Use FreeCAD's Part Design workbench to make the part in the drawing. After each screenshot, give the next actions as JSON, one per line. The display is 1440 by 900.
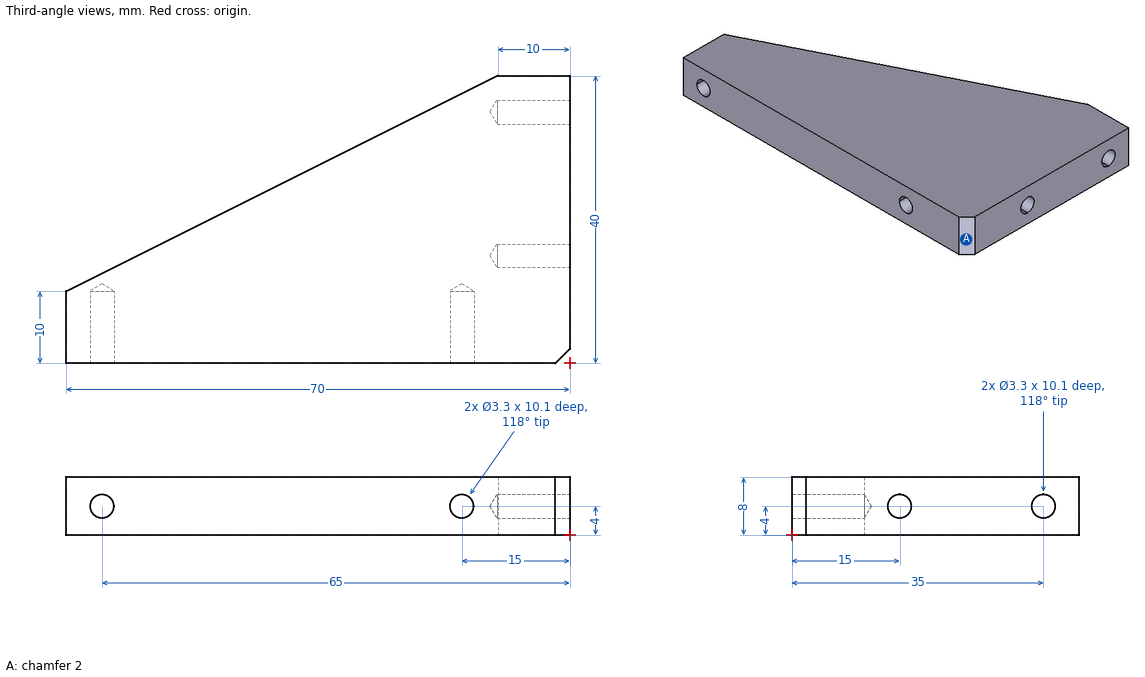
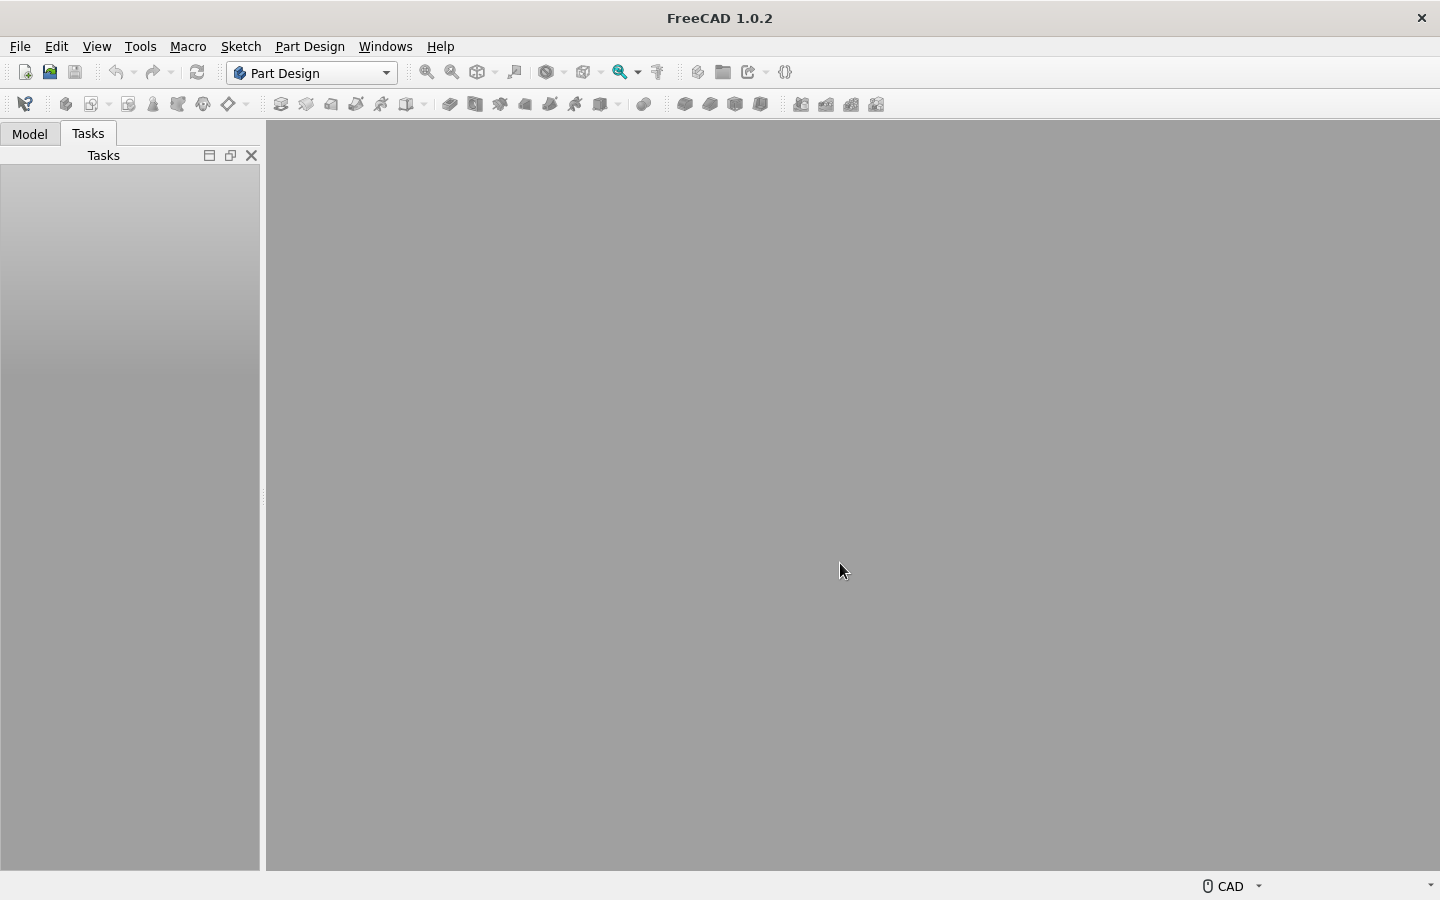
{"action": "key", "text": "ctrl+n"}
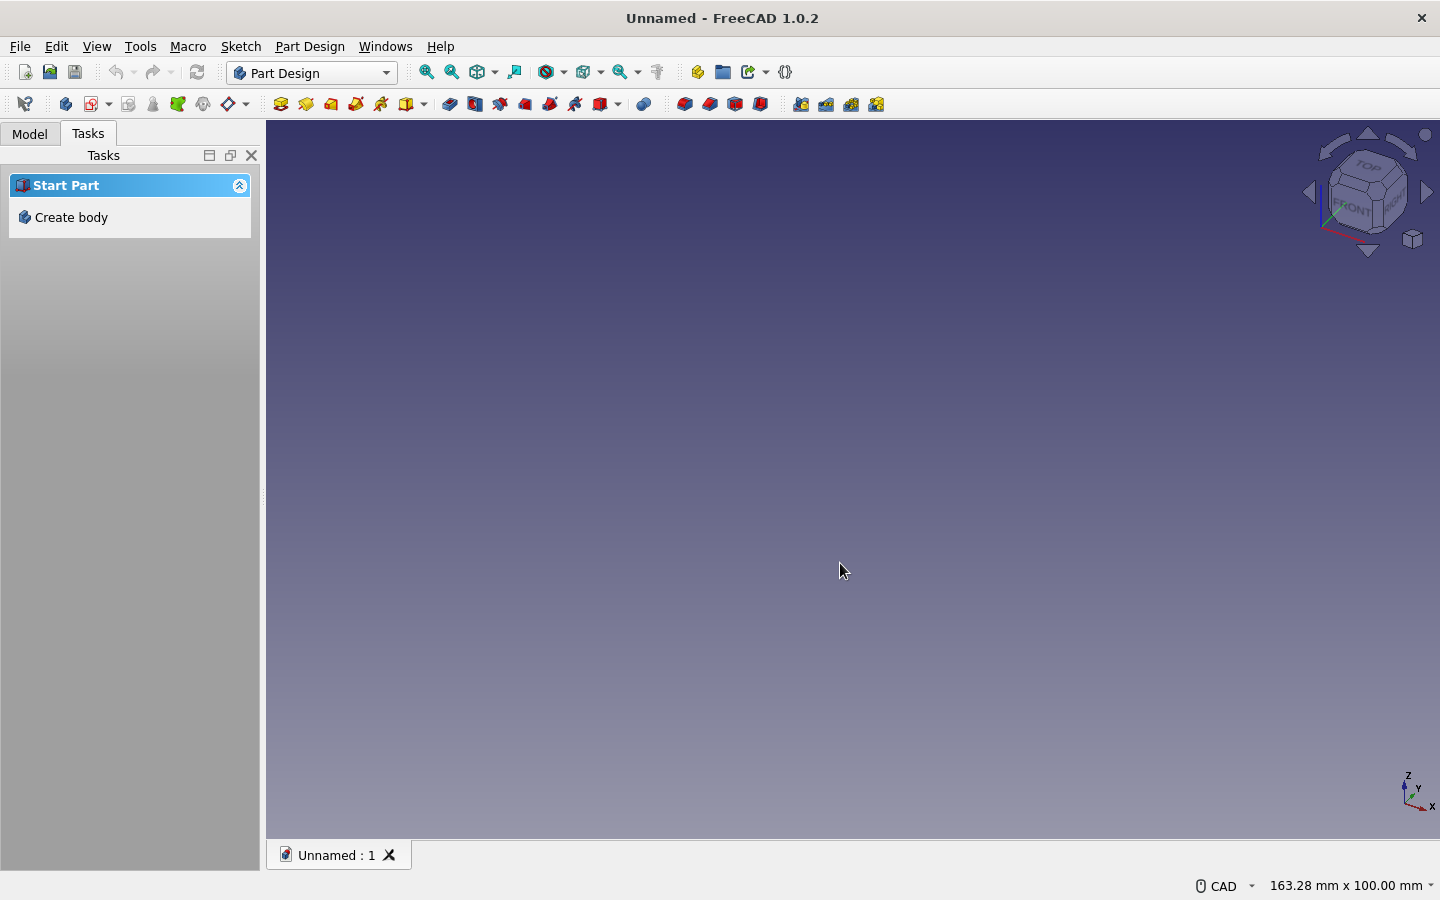
{"action": "left_click", "coordinate": [90, 104]}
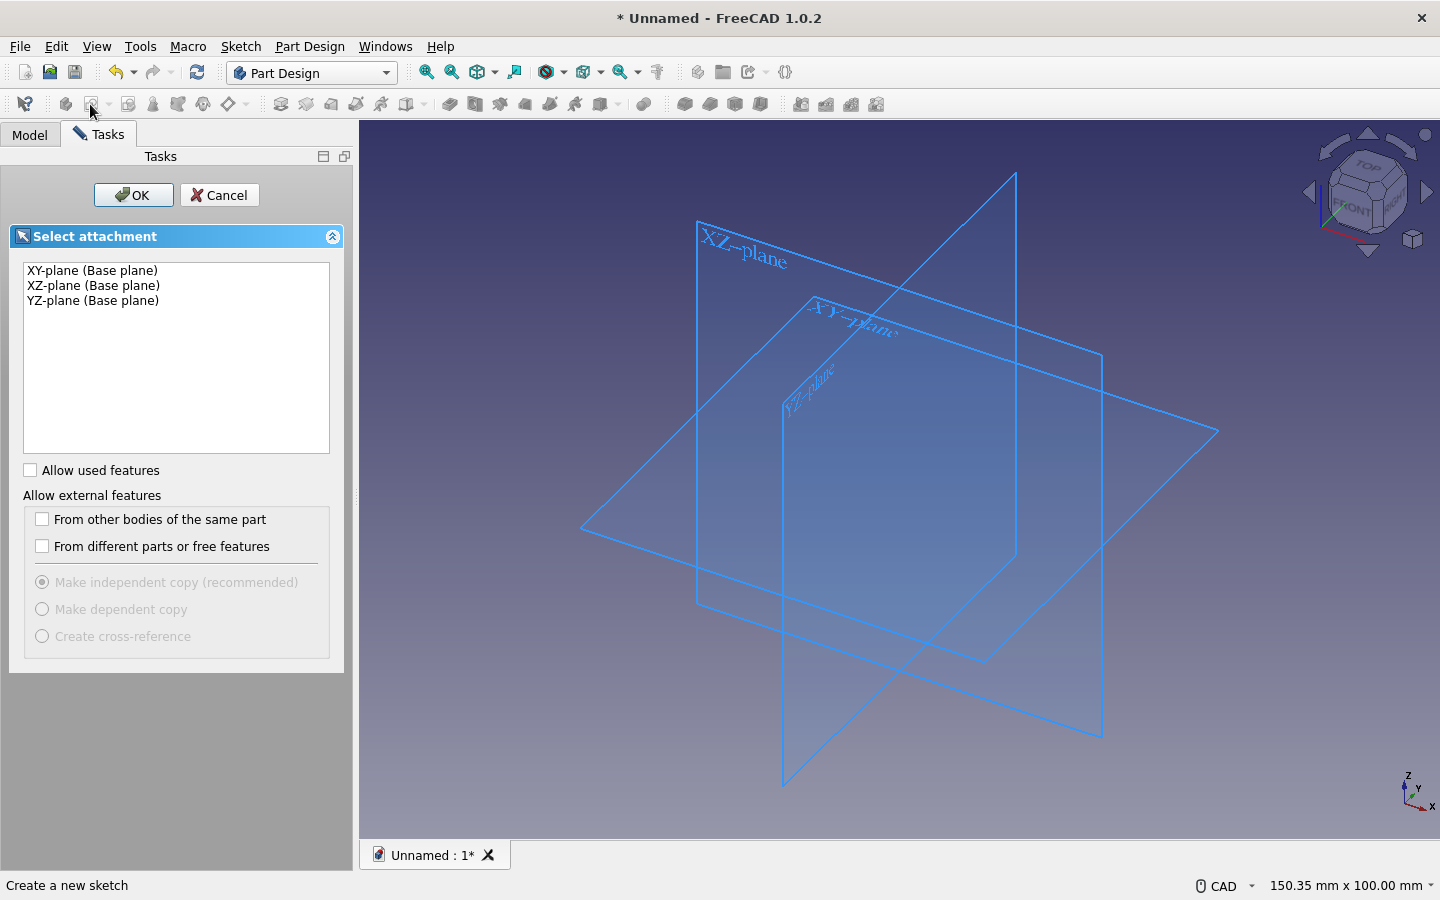
{"action": "left_click", "coordinate": [84, 270]}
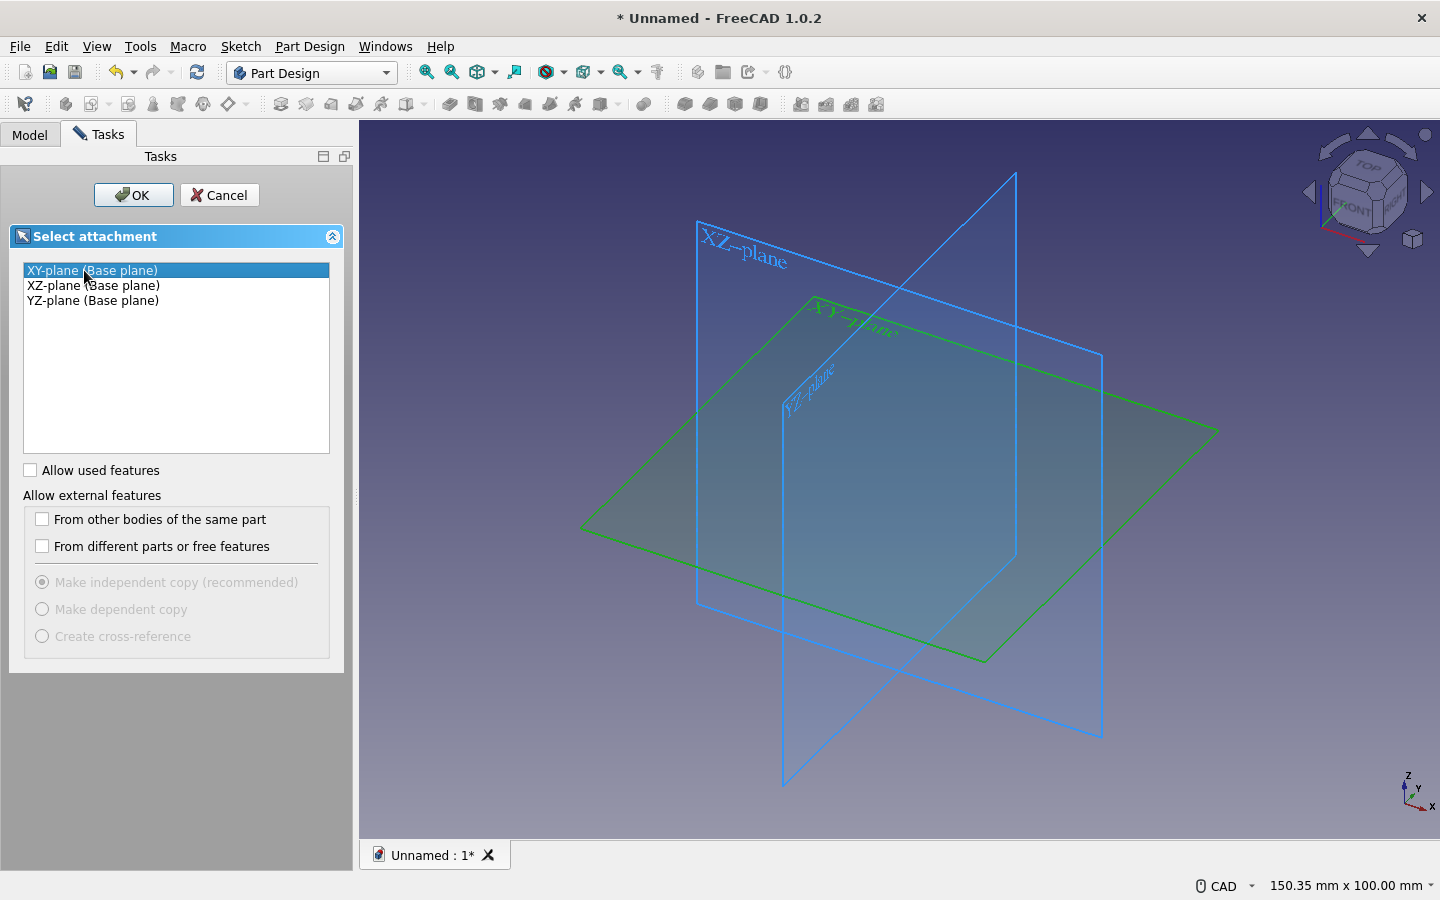
{"action": "left_click", "coordinate": [134, 195]}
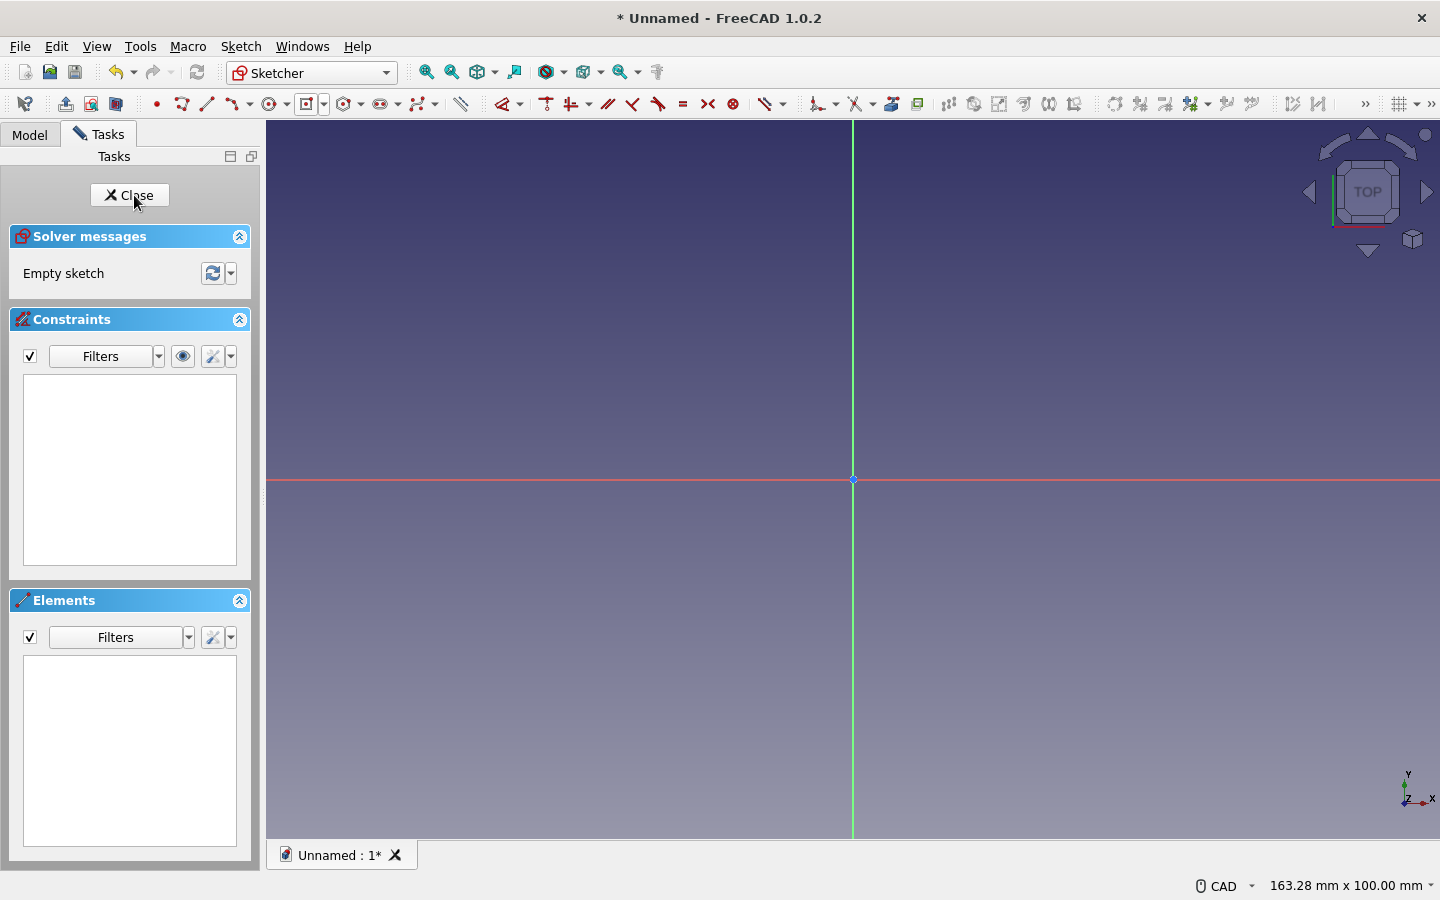
{"action": "scroll", "coordinate": [294, 148], "scroll_direction": "up", "scroll_amount": 2}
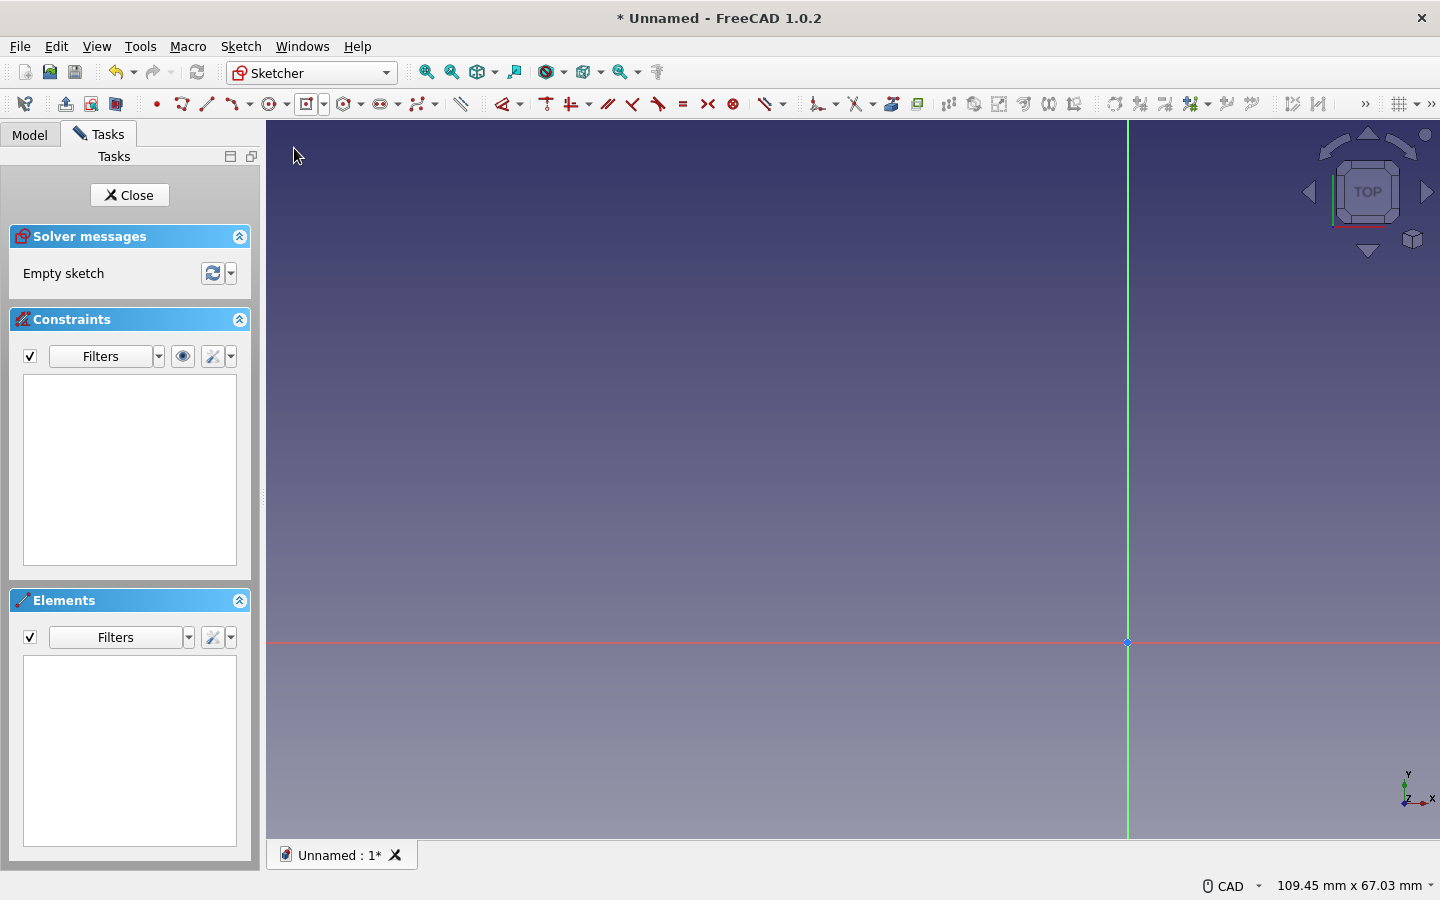
{"action": "left_click", "coordinate": [182, 104]}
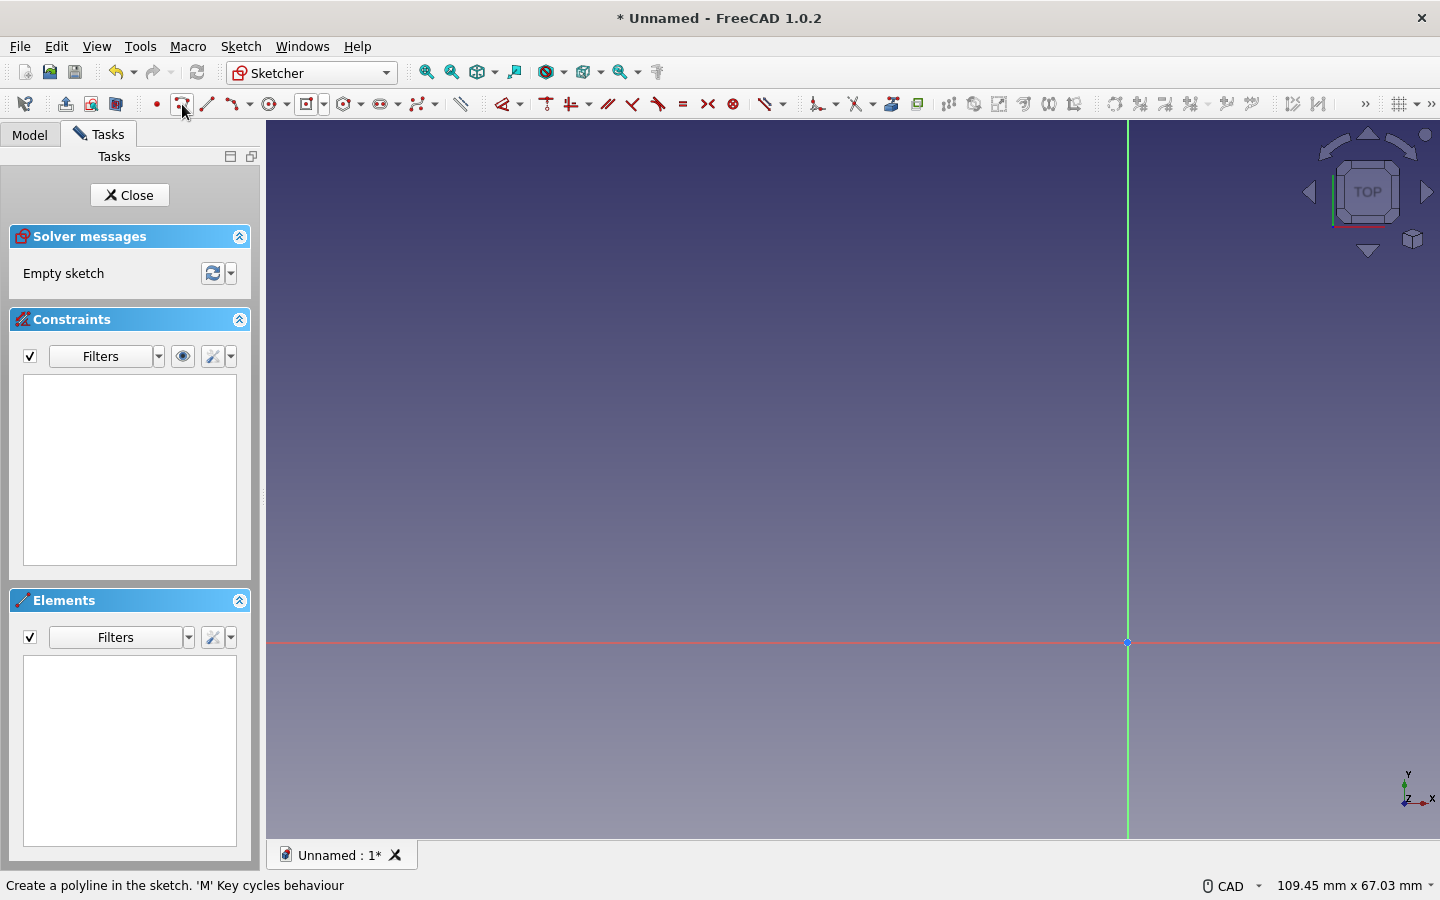
{"action": "left_click", "coordinate": [1128, 643]}
{"action": "left_click", "coordinate": [1119, 213]}
{"action": "left_click", "coordinate": [1021, 213]}
{"action": "left_click", "coordinate": [377, 535]}
{"action": "left_click", "coordinate": [377, 634]}
{"action": "left_click", "coordinate": [1128, 643]}
{"action": "key", "text": "Escape"}
{"action": "key", "text": "Escape"}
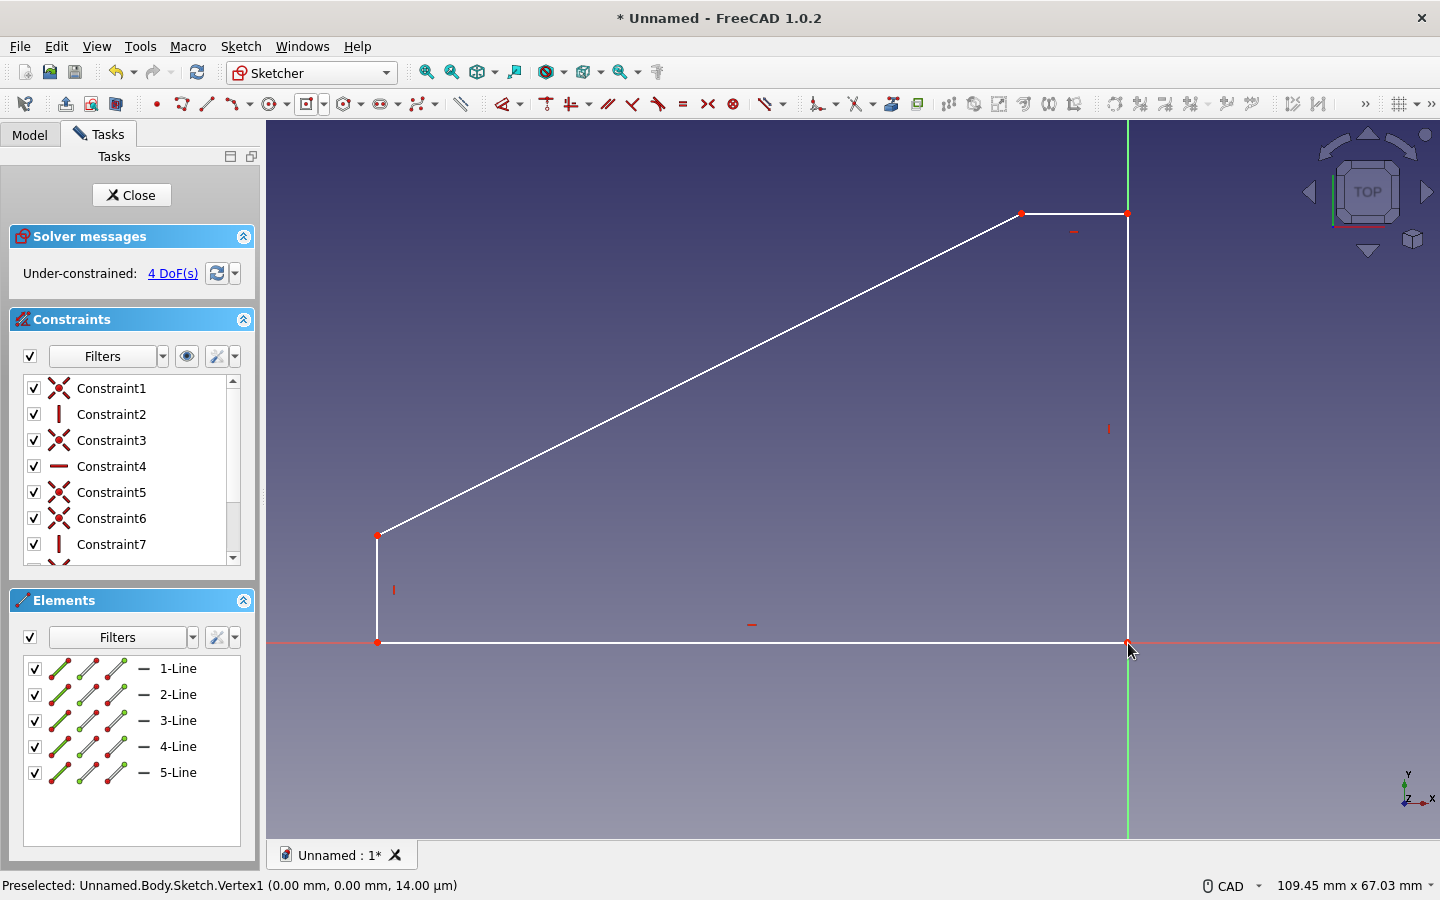
{"action": "left_click", "coordinate": [502, 104]}